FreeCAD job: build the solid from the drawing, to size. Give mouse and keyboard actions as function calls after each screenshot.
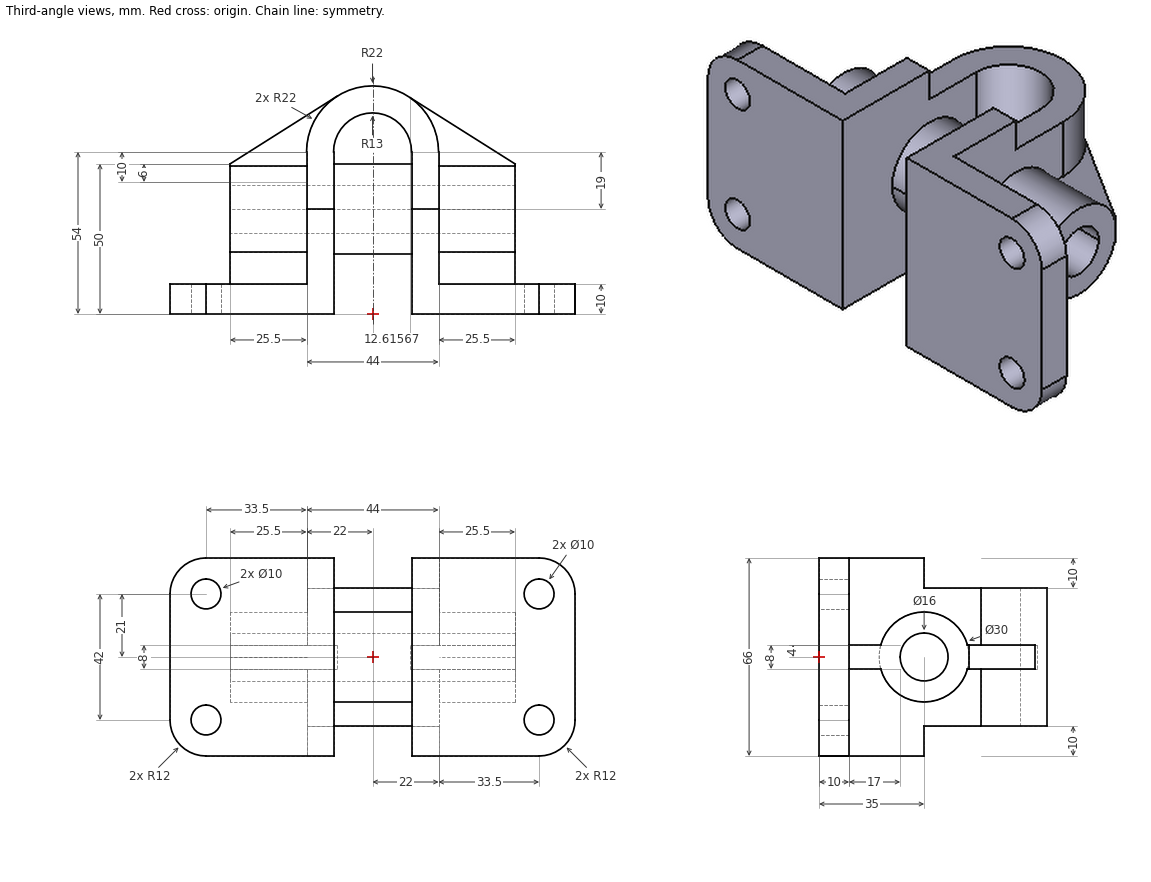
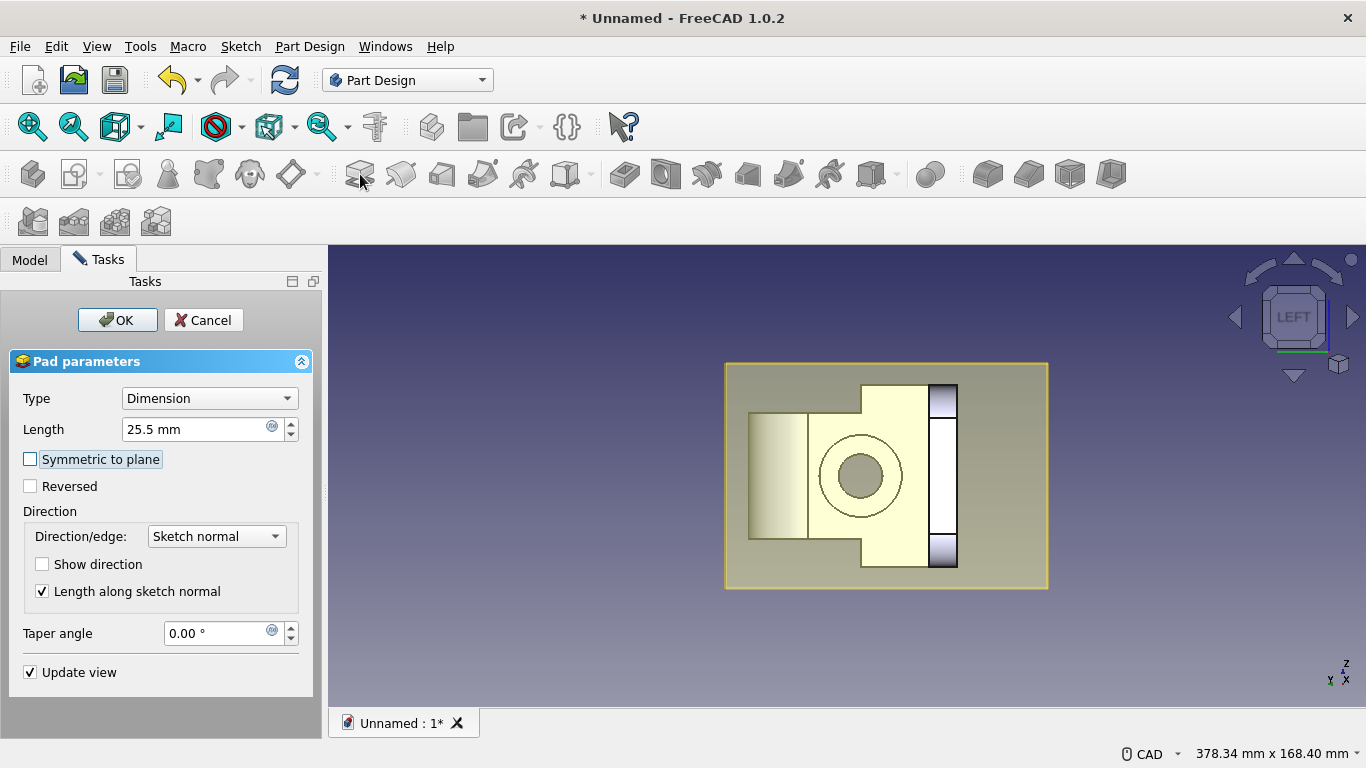
click(118, 320)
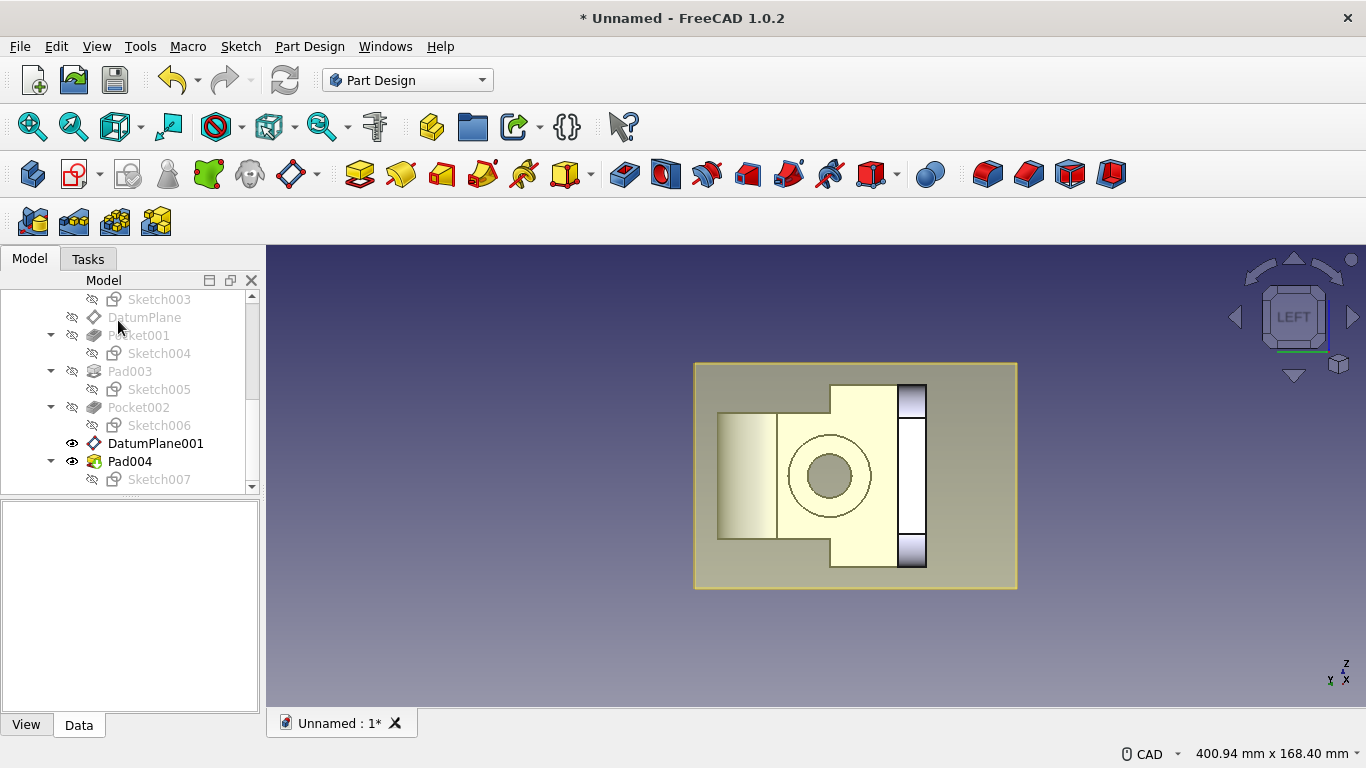
click(117, 443)
key(space)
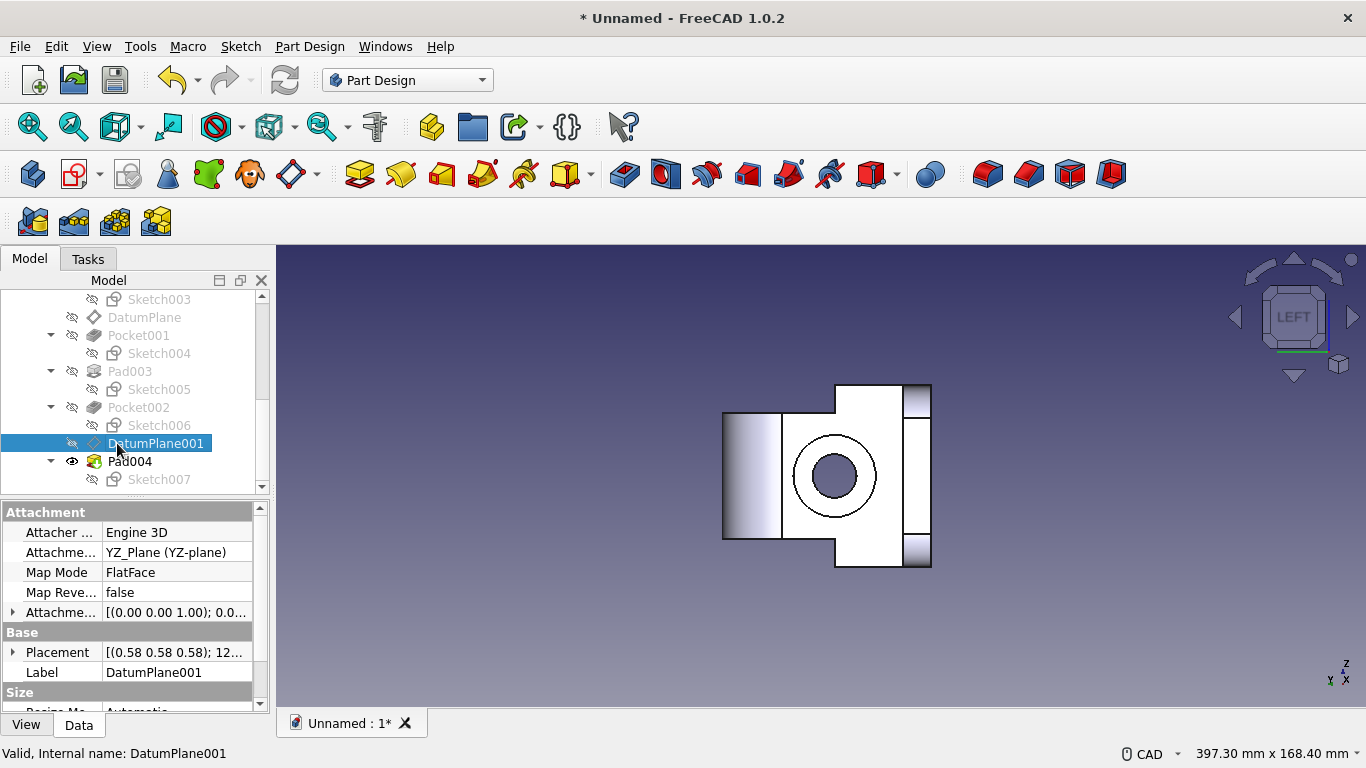
click(33, 128)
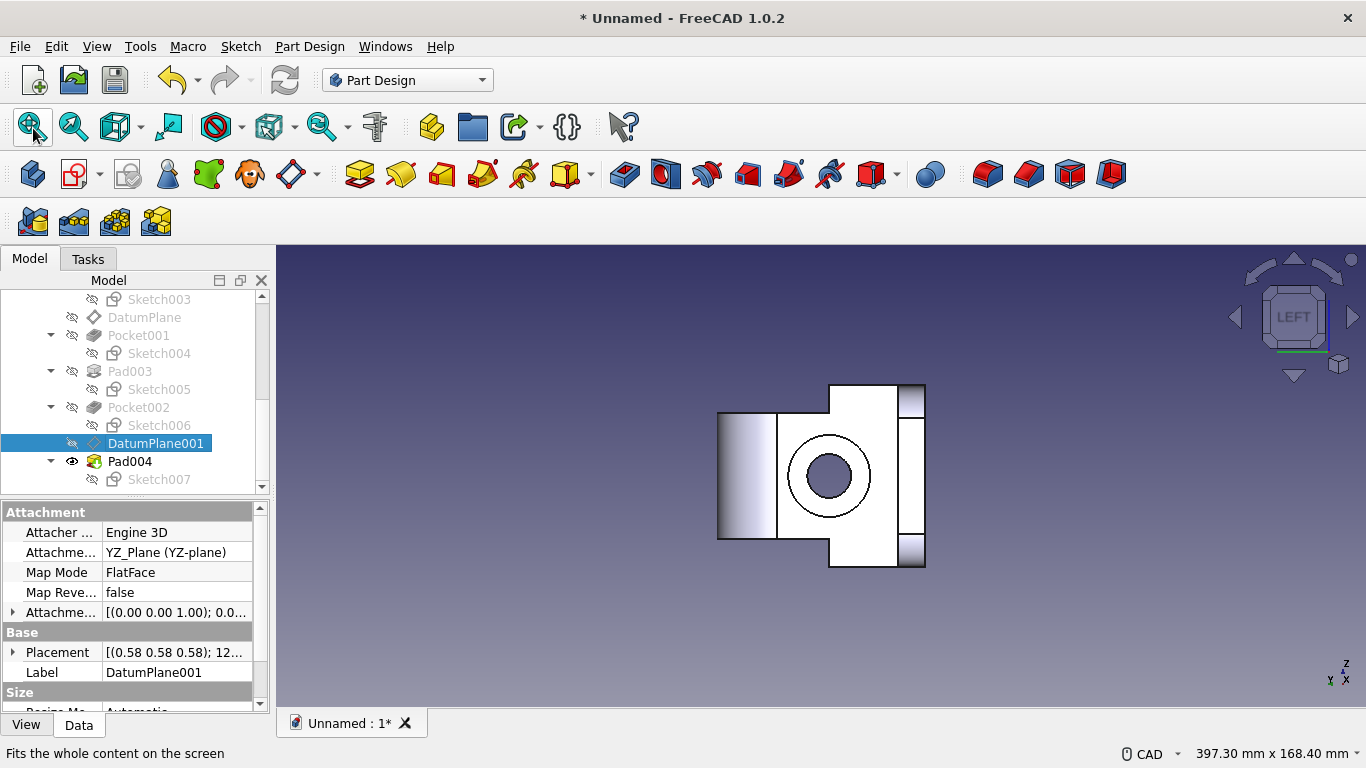
key(0)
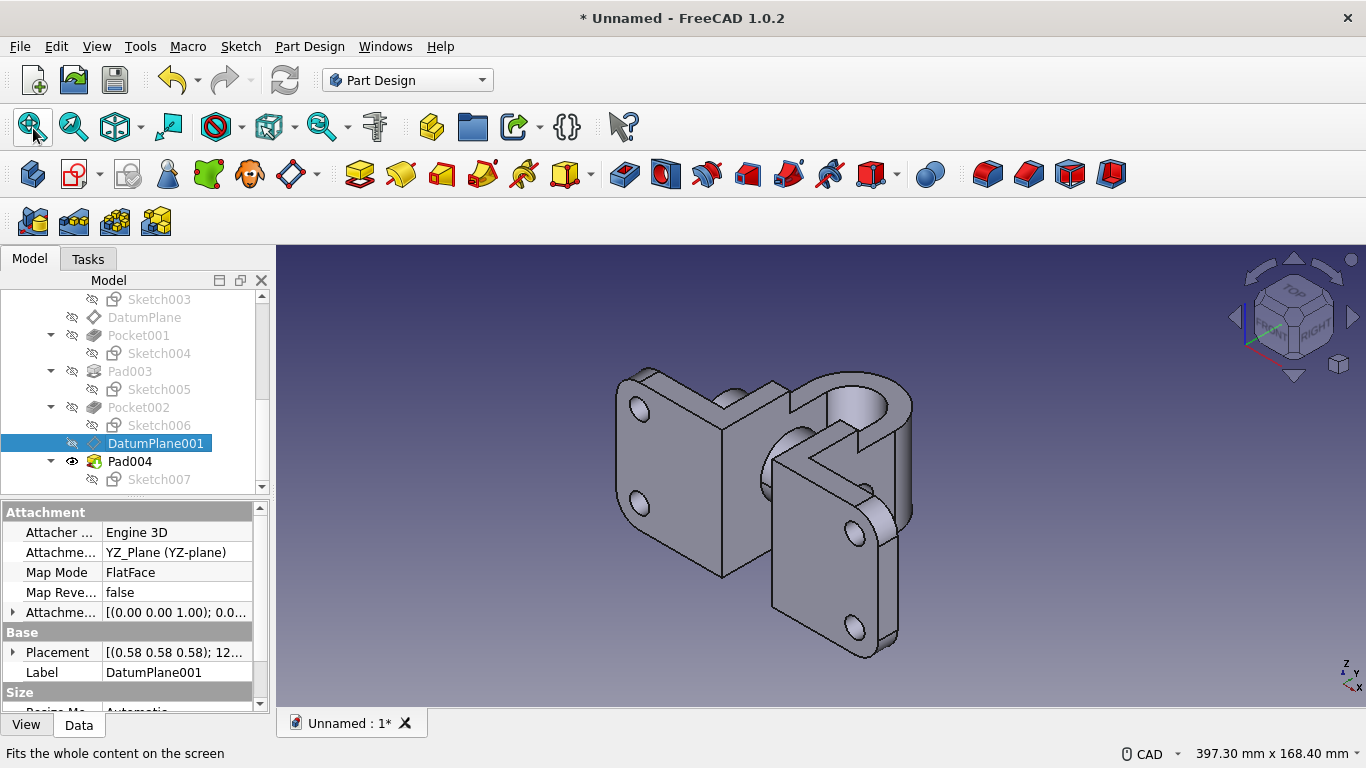
click(876, 471)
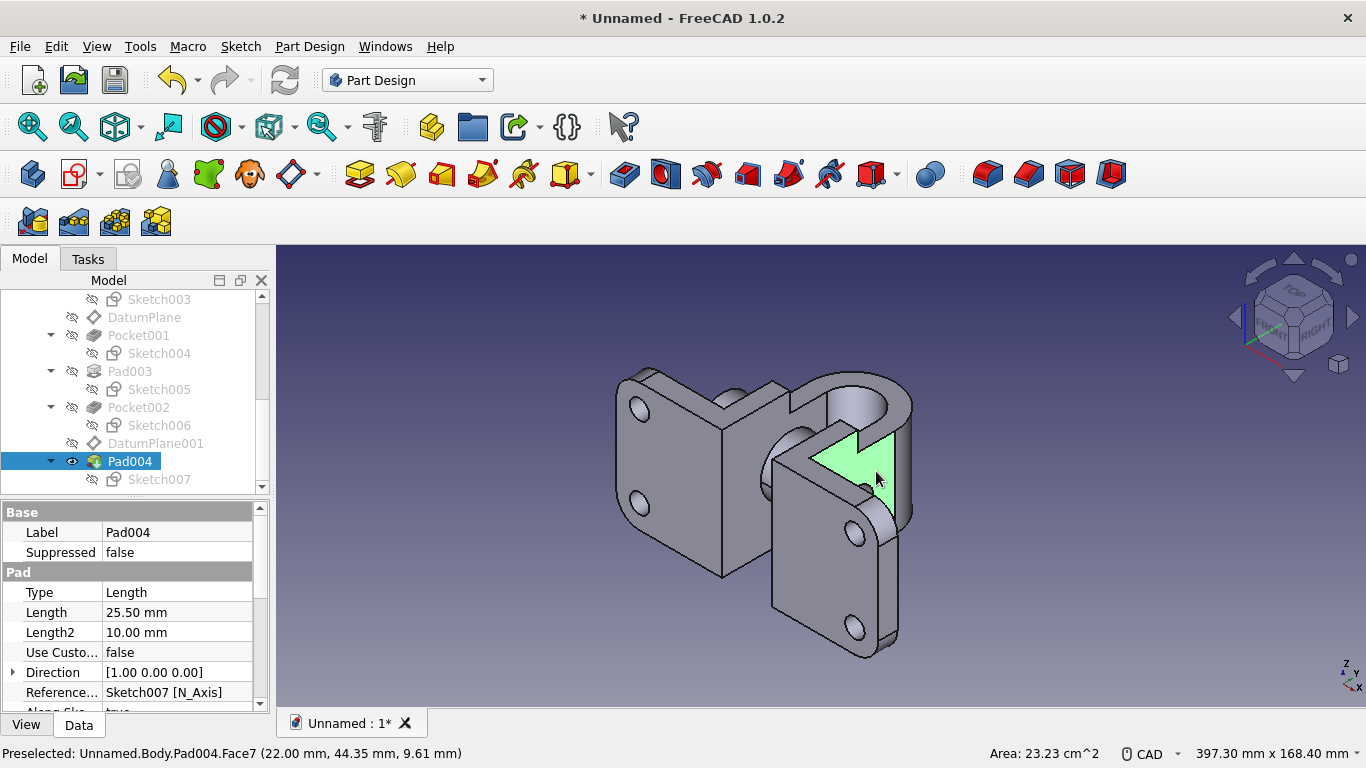
click(74, 174)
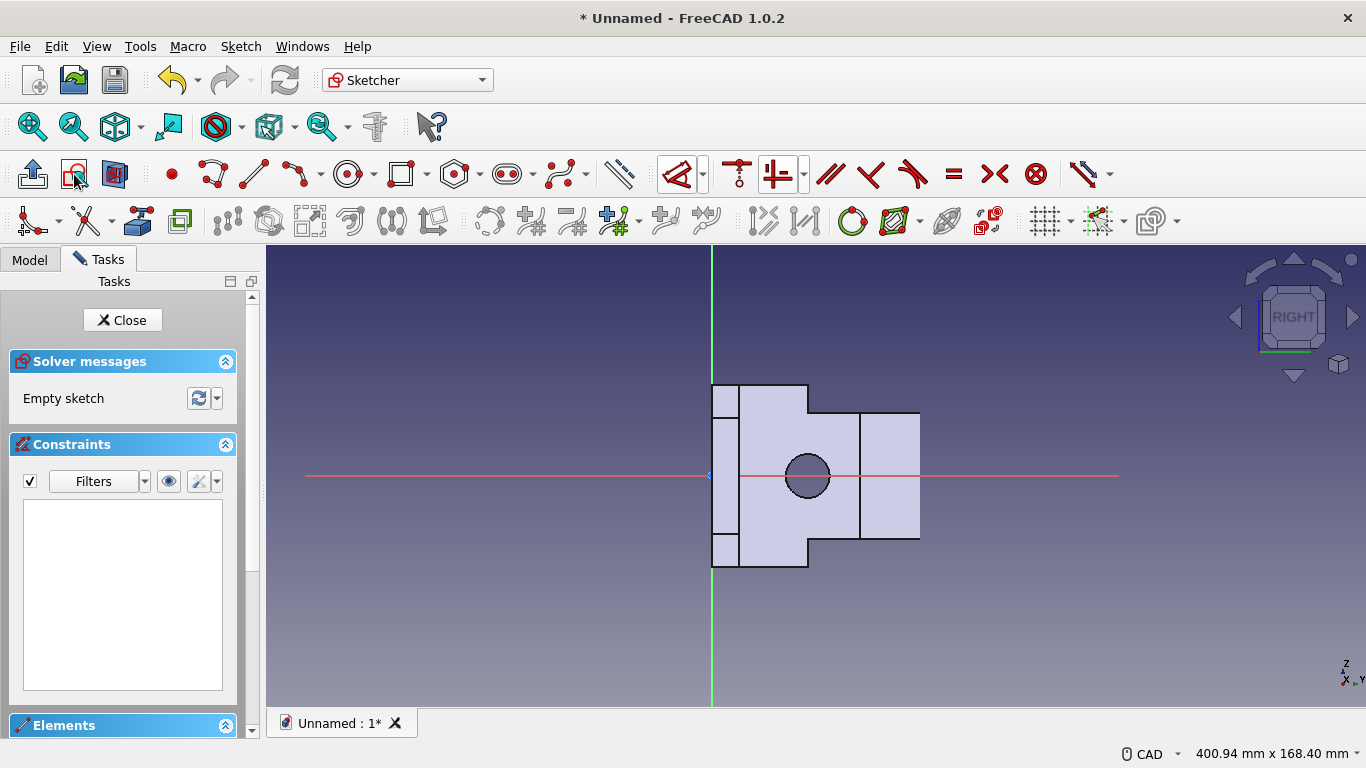
scroll(794, 476, up, 6)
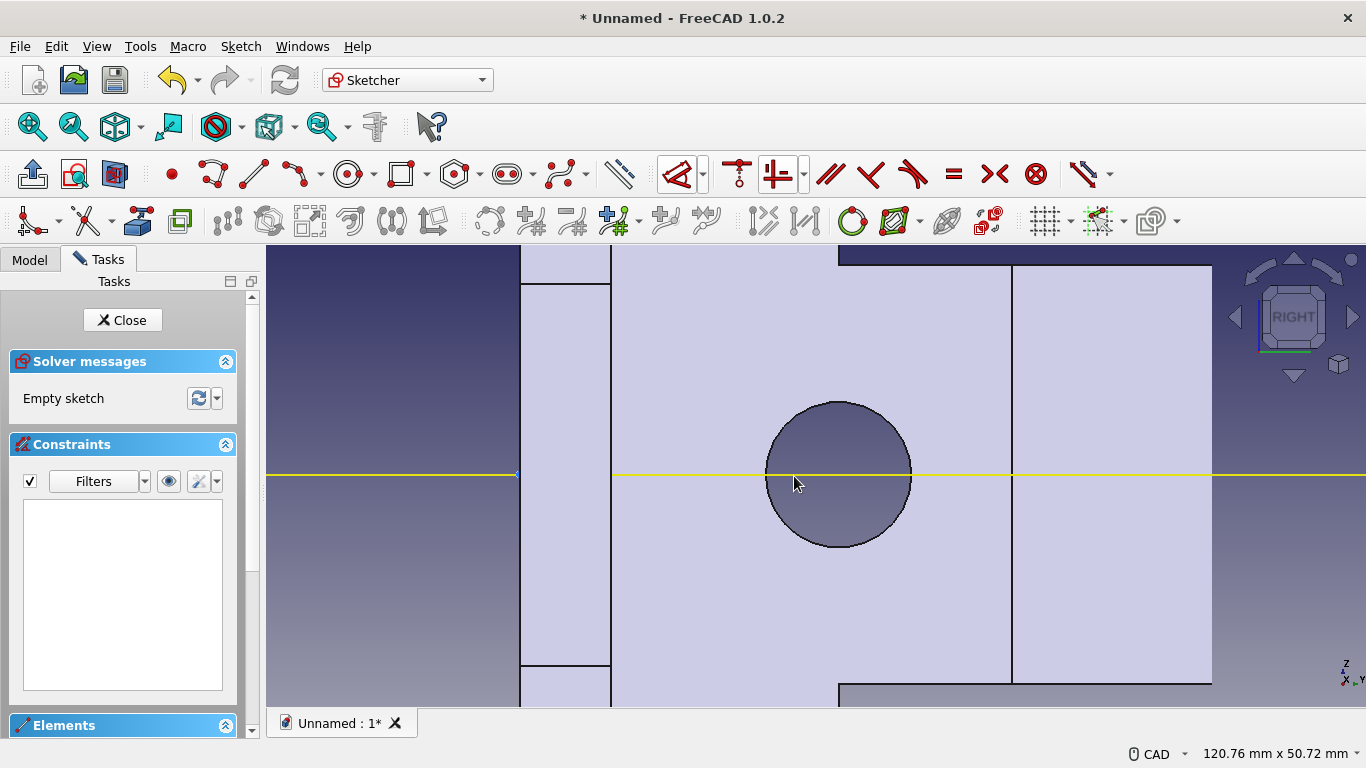
click(348, 174)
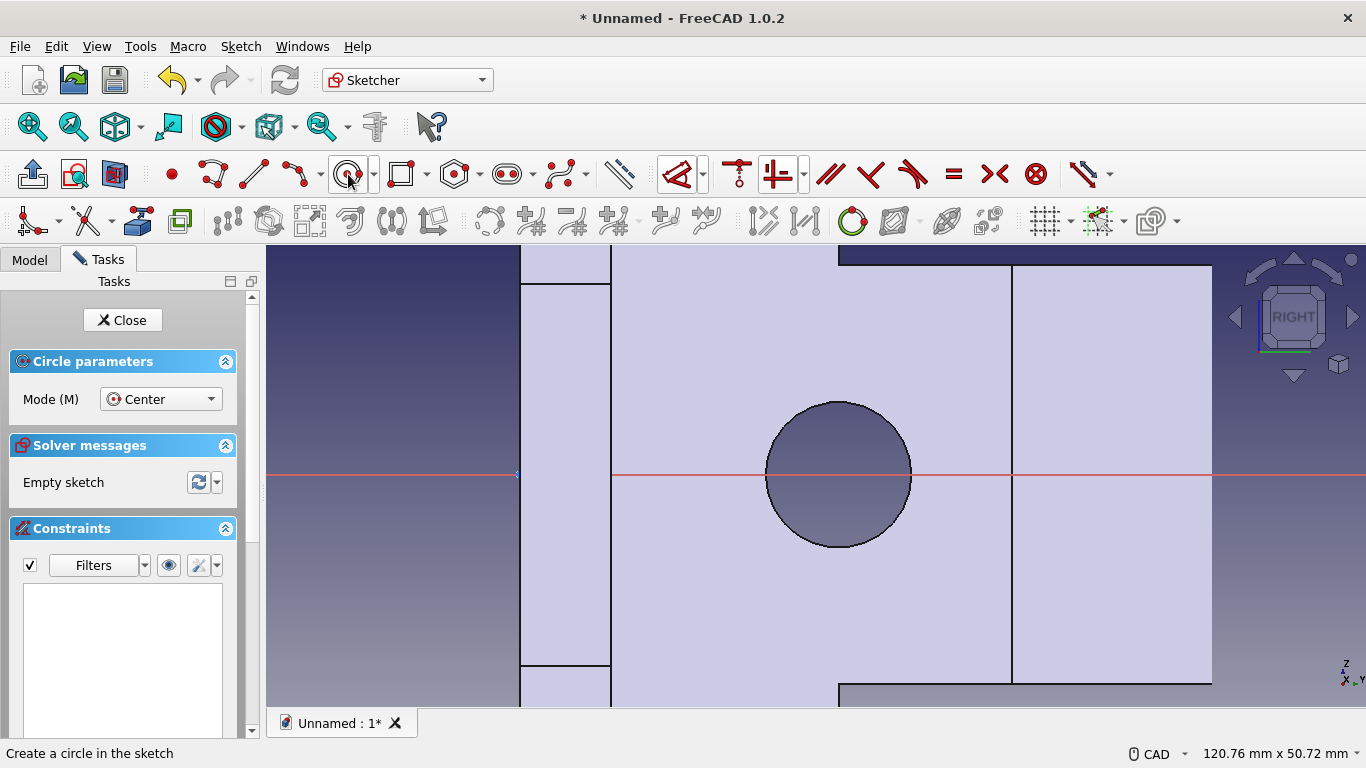
click(839, 475)
move(935, 378)